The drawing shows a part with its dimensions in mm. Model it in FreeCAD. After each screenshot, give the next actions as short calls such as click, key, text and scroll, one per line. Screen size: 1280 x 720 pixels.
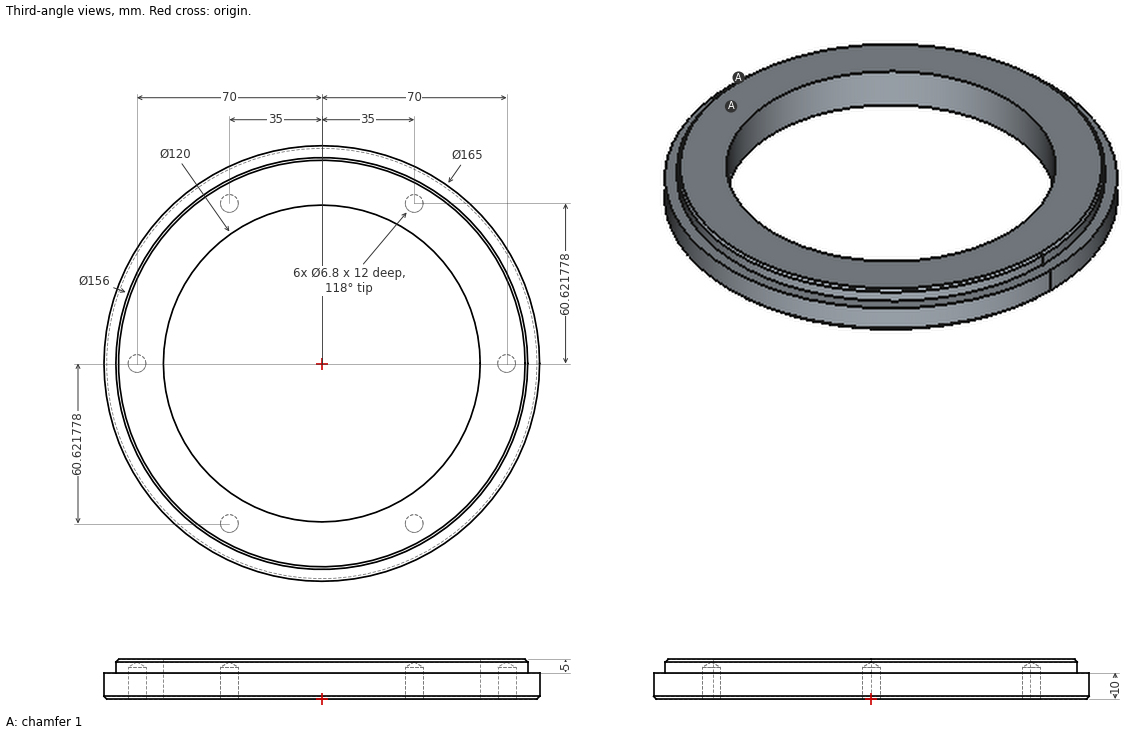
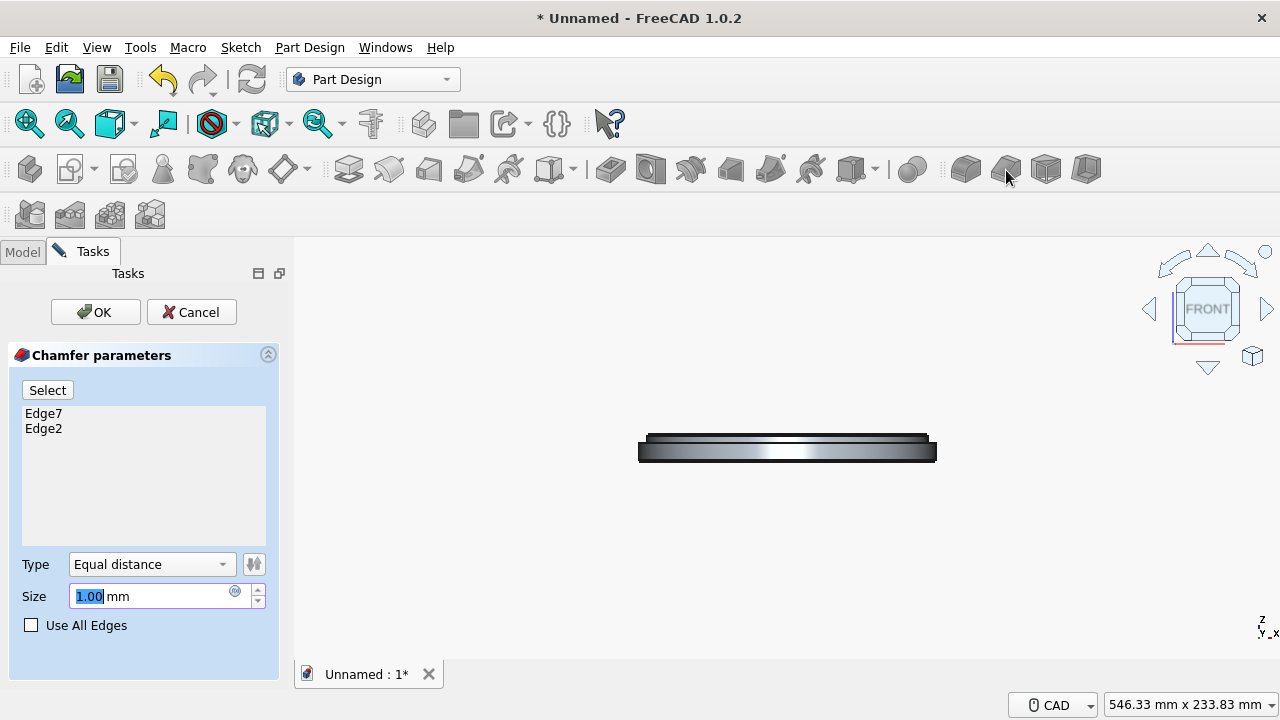
text(1)
key(Tab)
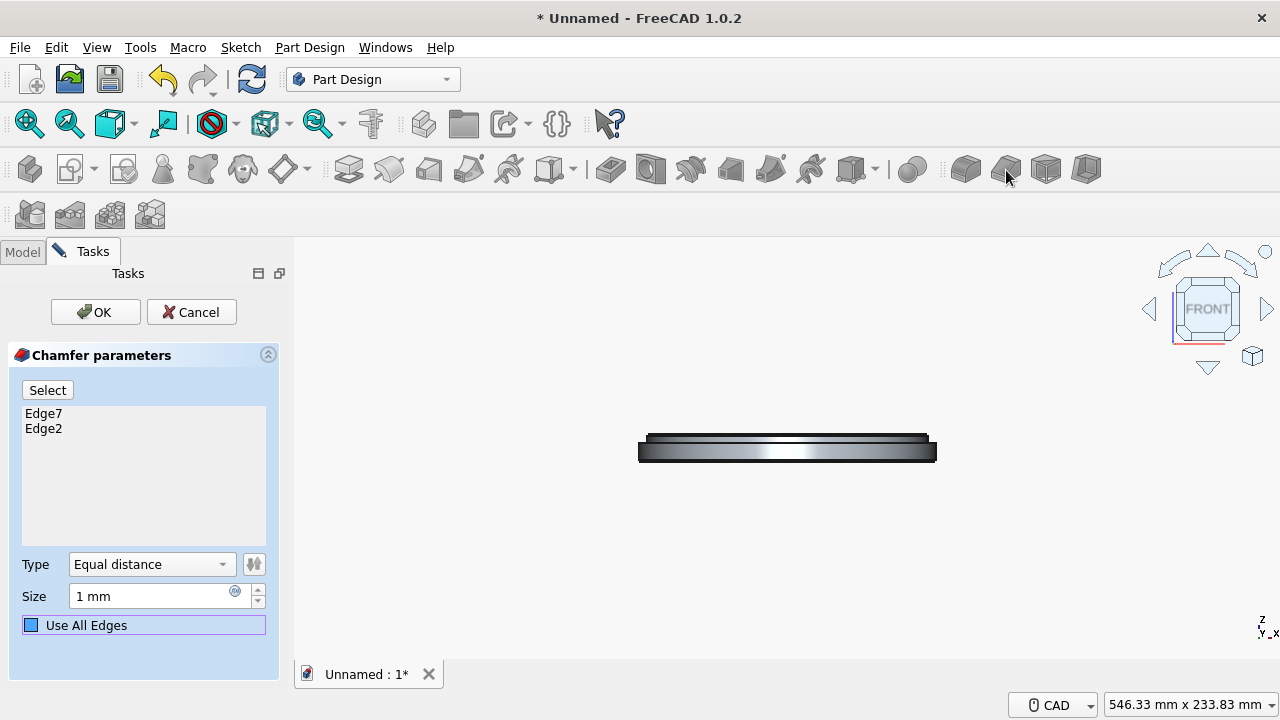
click(96, 312)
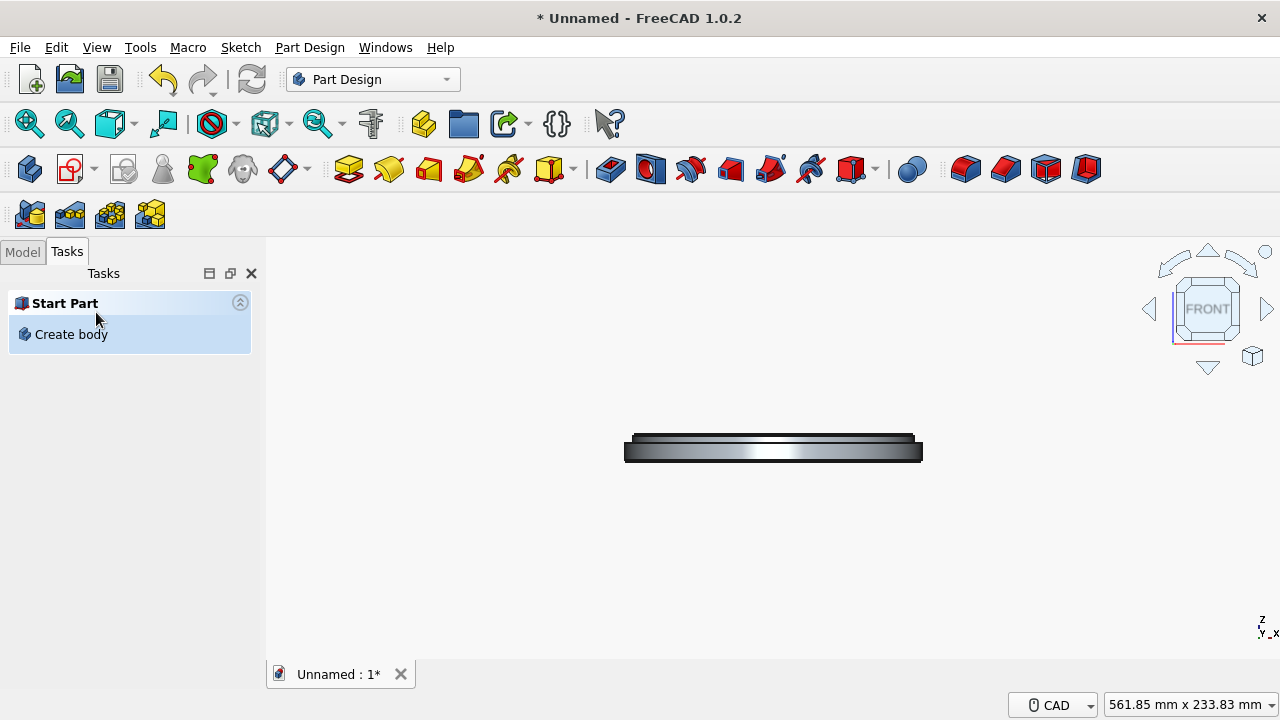
click(30, 124)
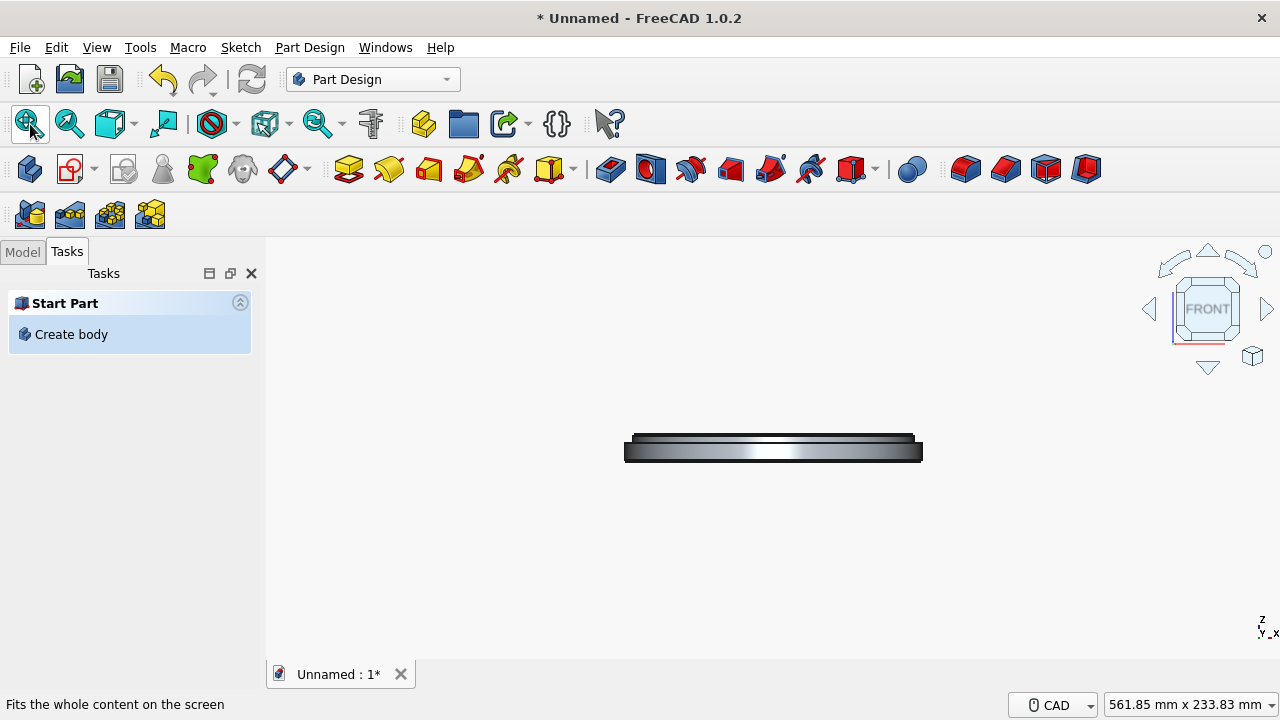
click(70, 170)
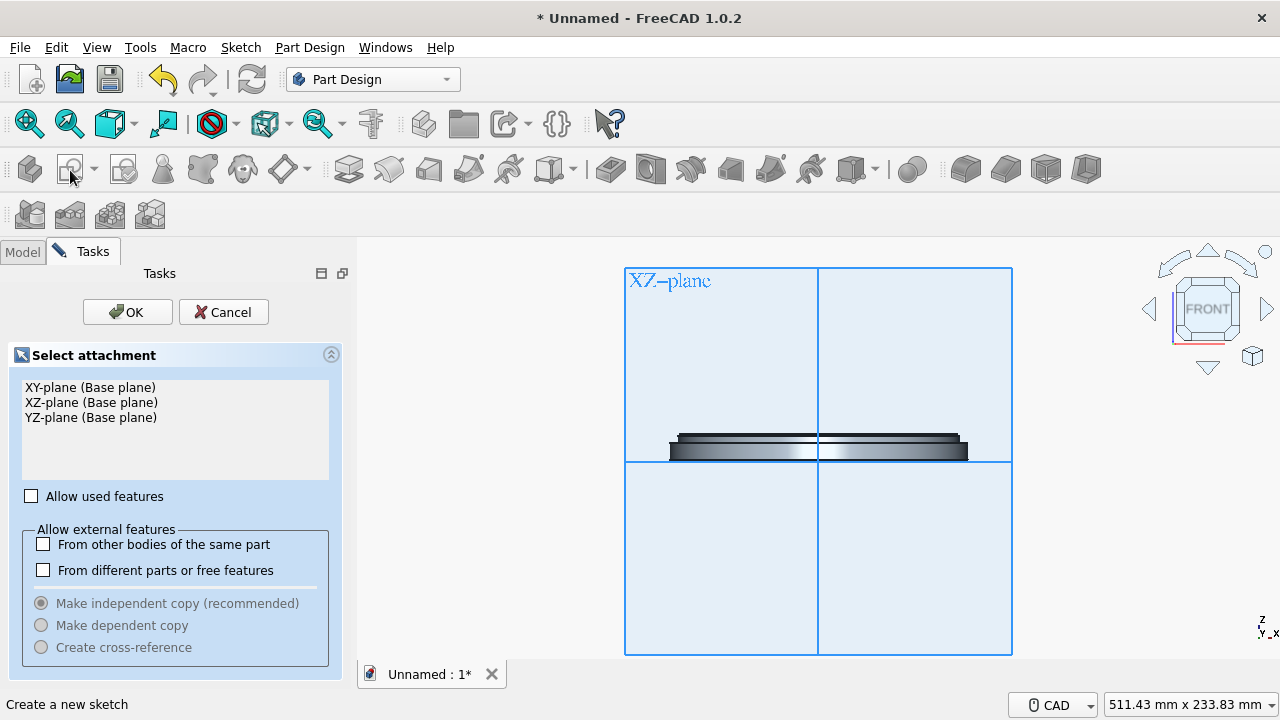
click(82, 388)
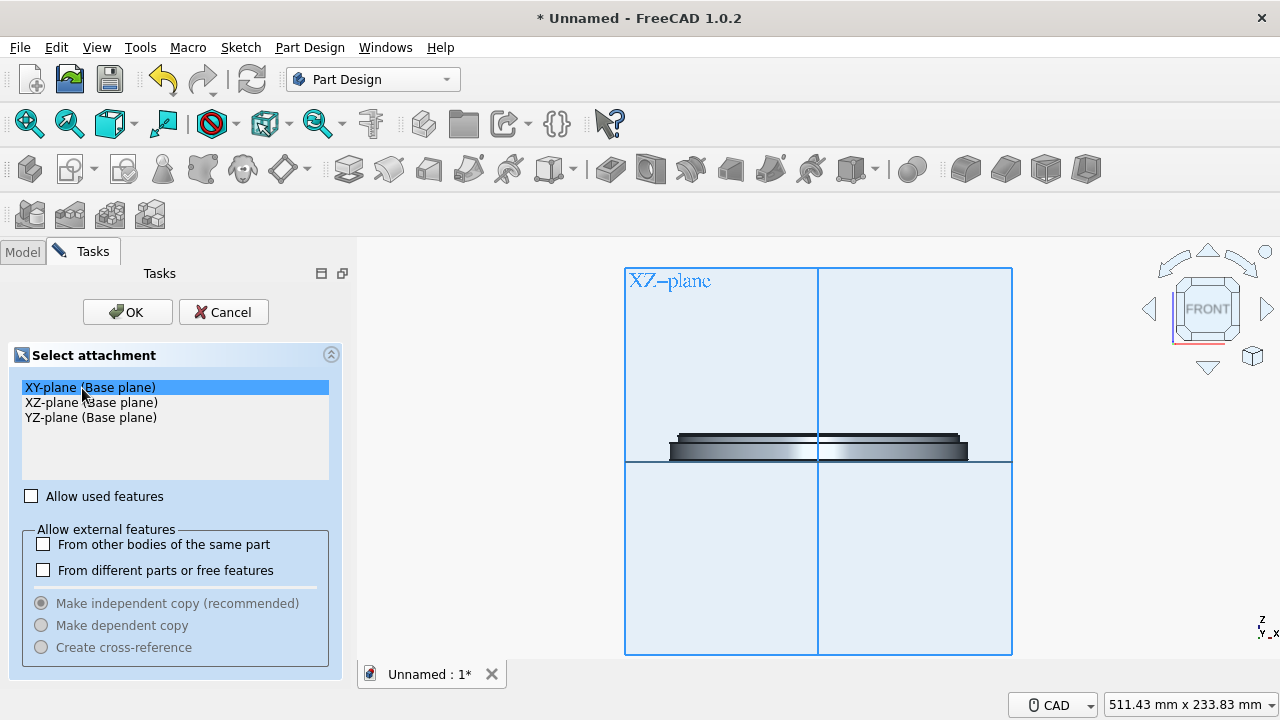
click(128, 312)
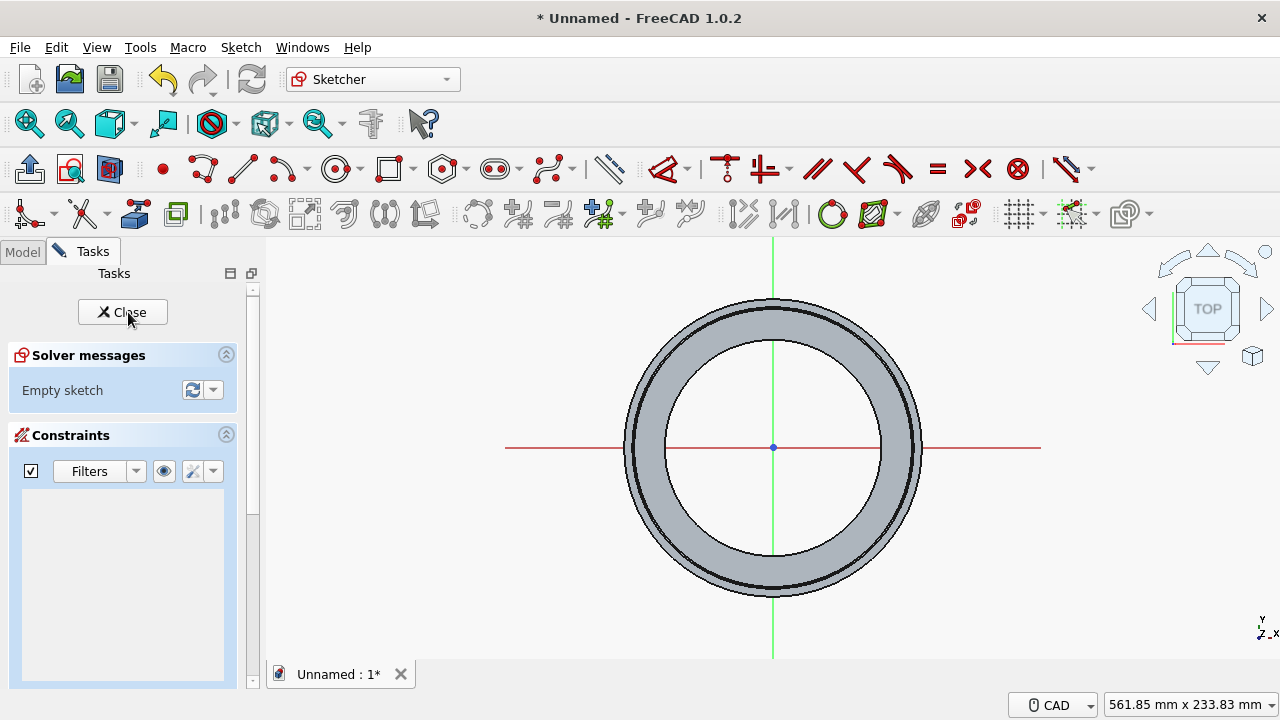
click(110, 170)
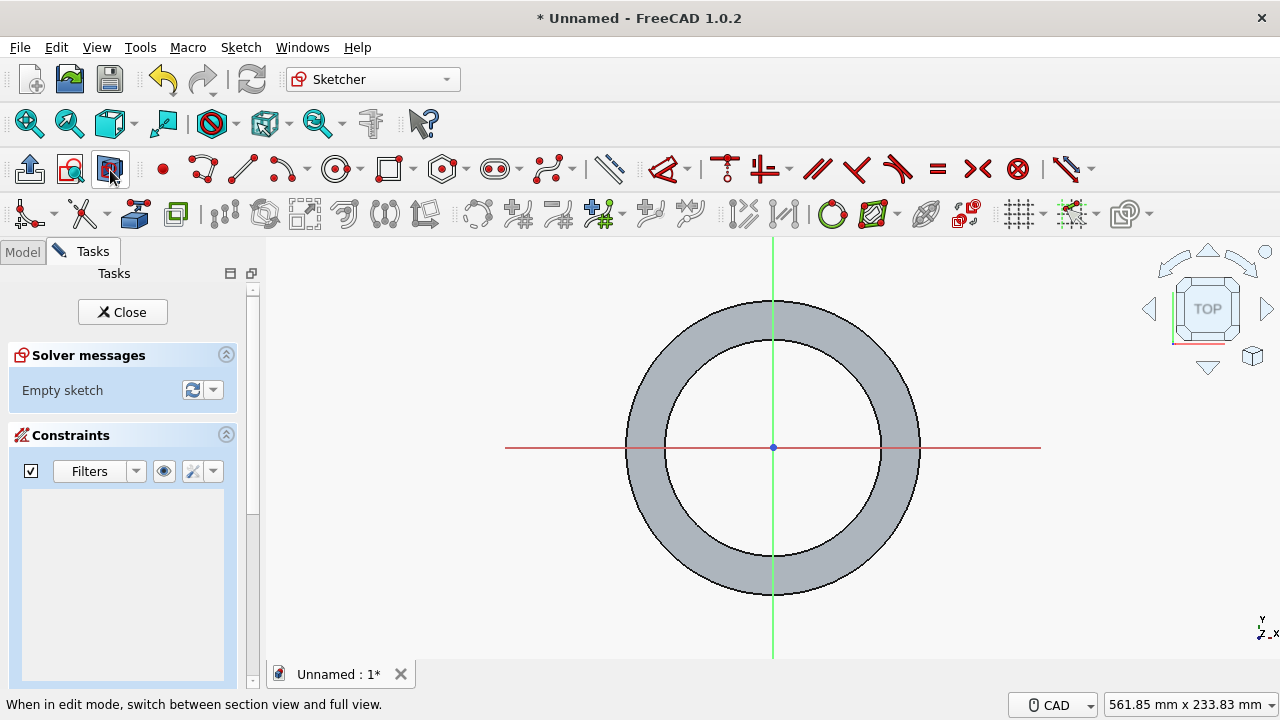
click(336, 170)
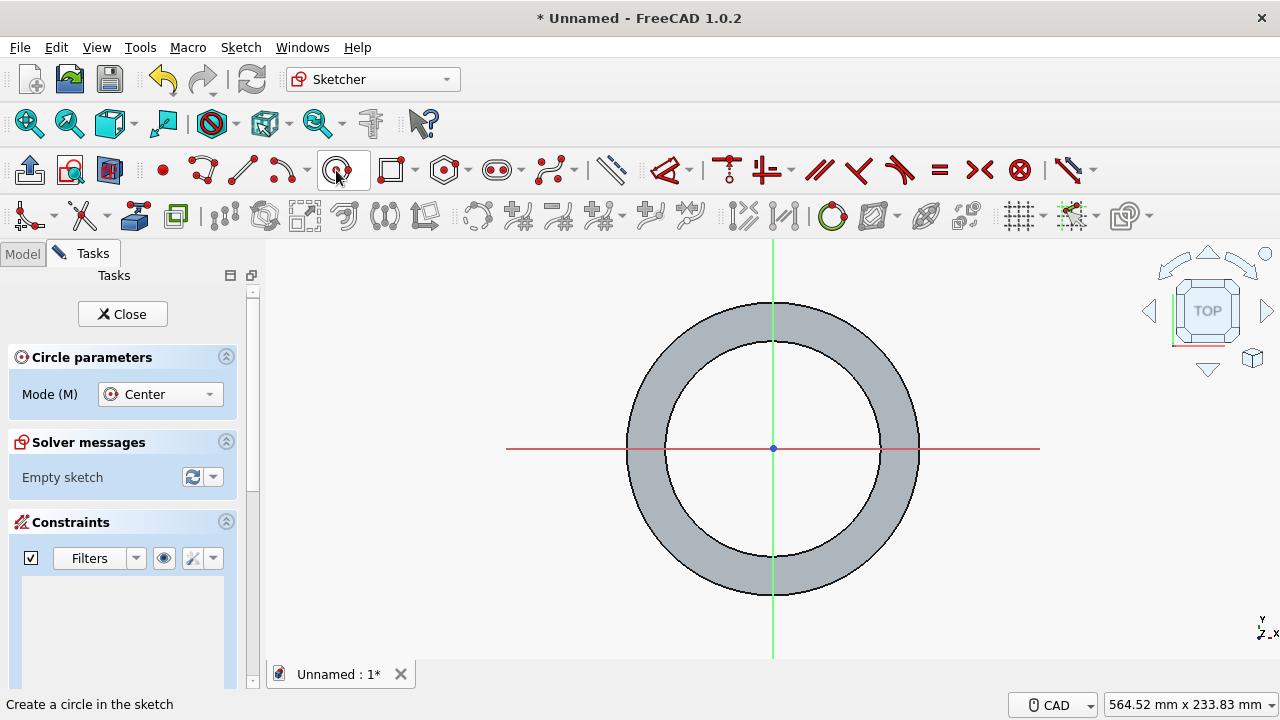
scroll(836, 340, up, 7)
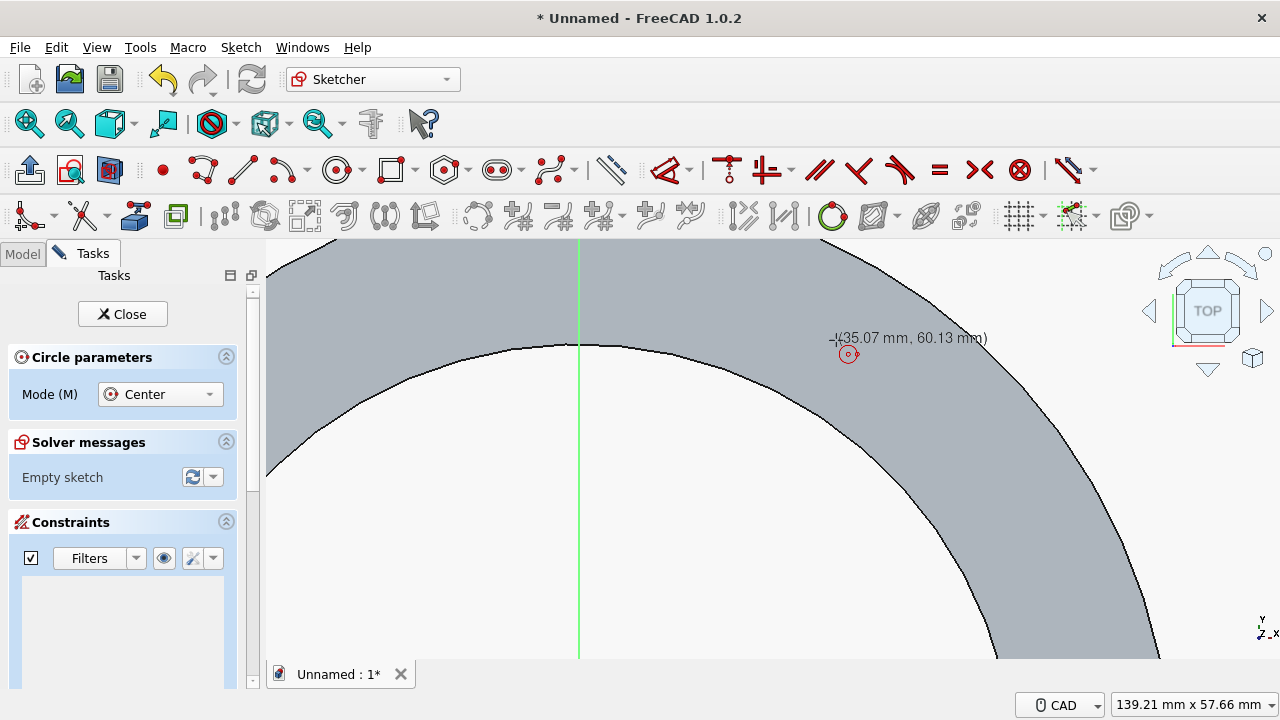
scroll(759, 306, down, 6)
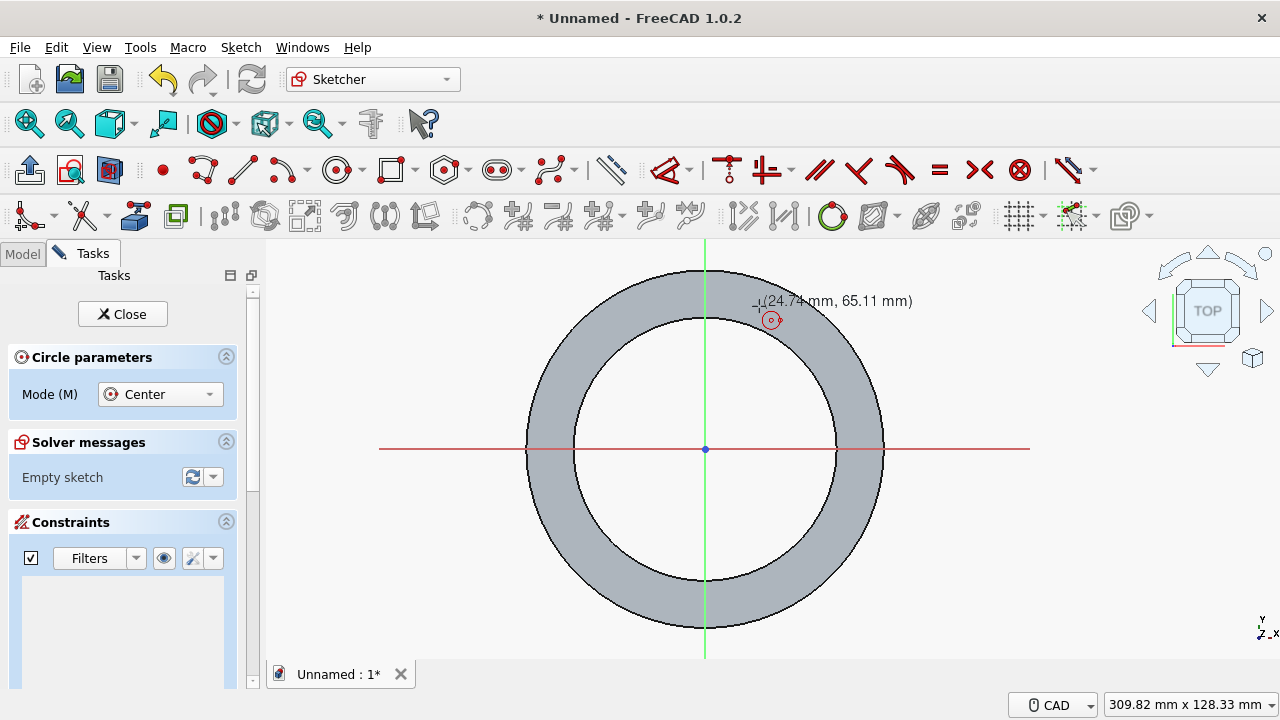
click(782, 316)
move(787, 311)